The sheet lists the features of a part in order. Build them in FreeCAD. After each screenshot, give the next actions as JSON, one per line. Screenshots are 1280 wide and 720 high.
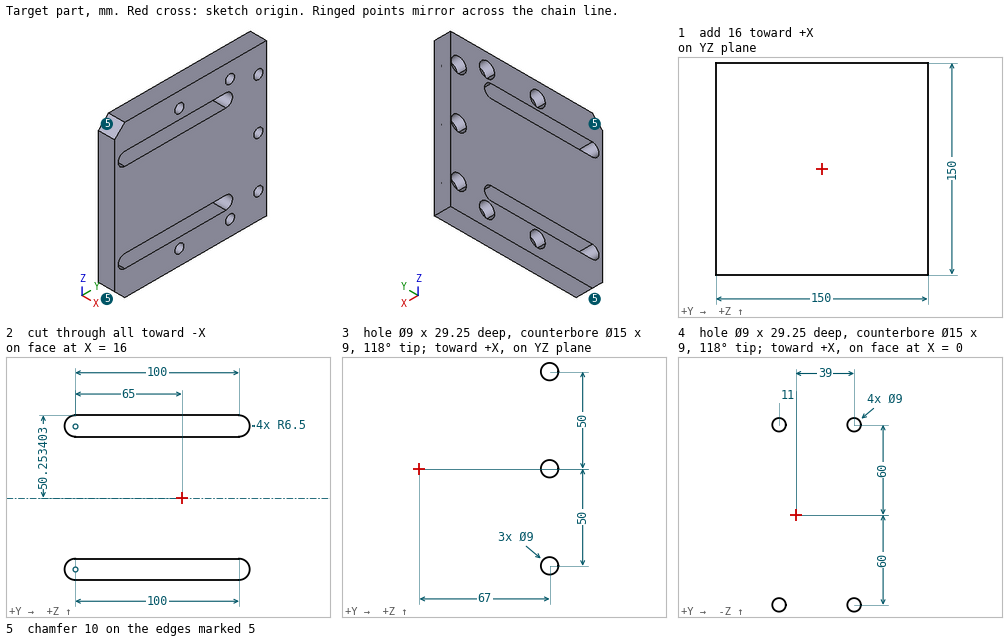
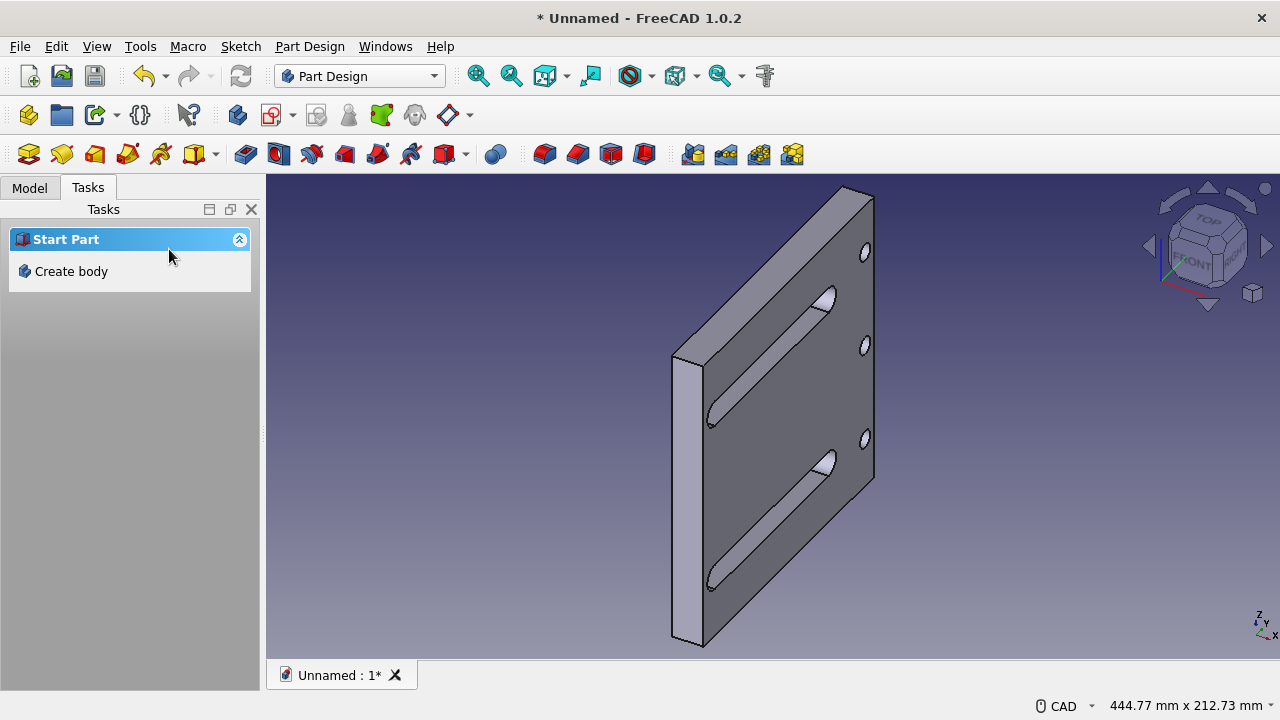
{"action": "key", "text": "6"}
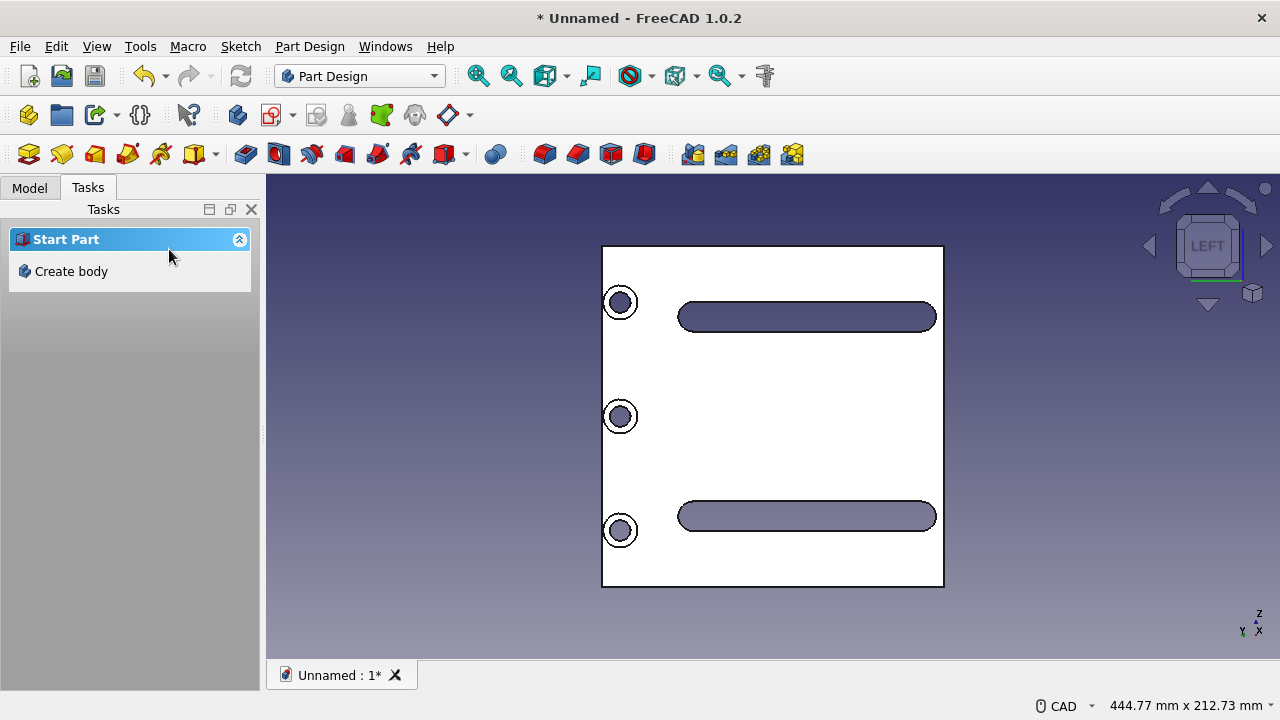
{"action": "left_click", "coordinate": [773, 416]}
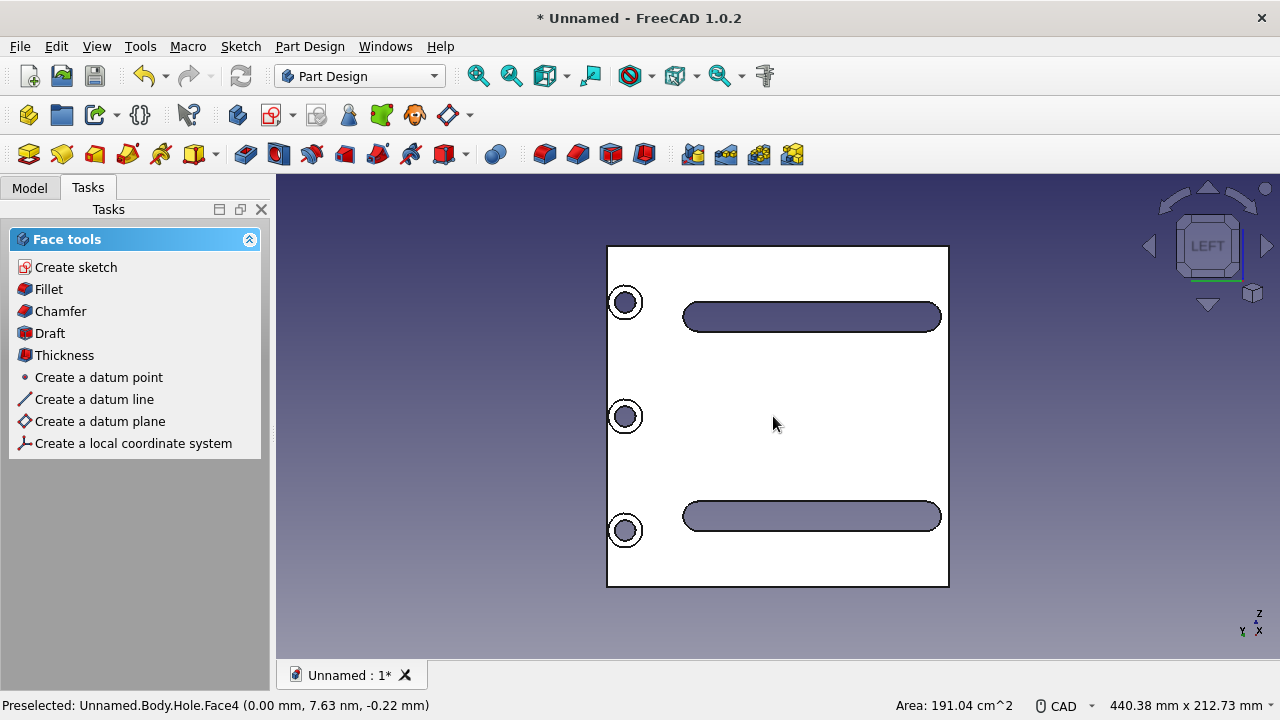
{"action": "left_click", "coordinate": [270, 116]}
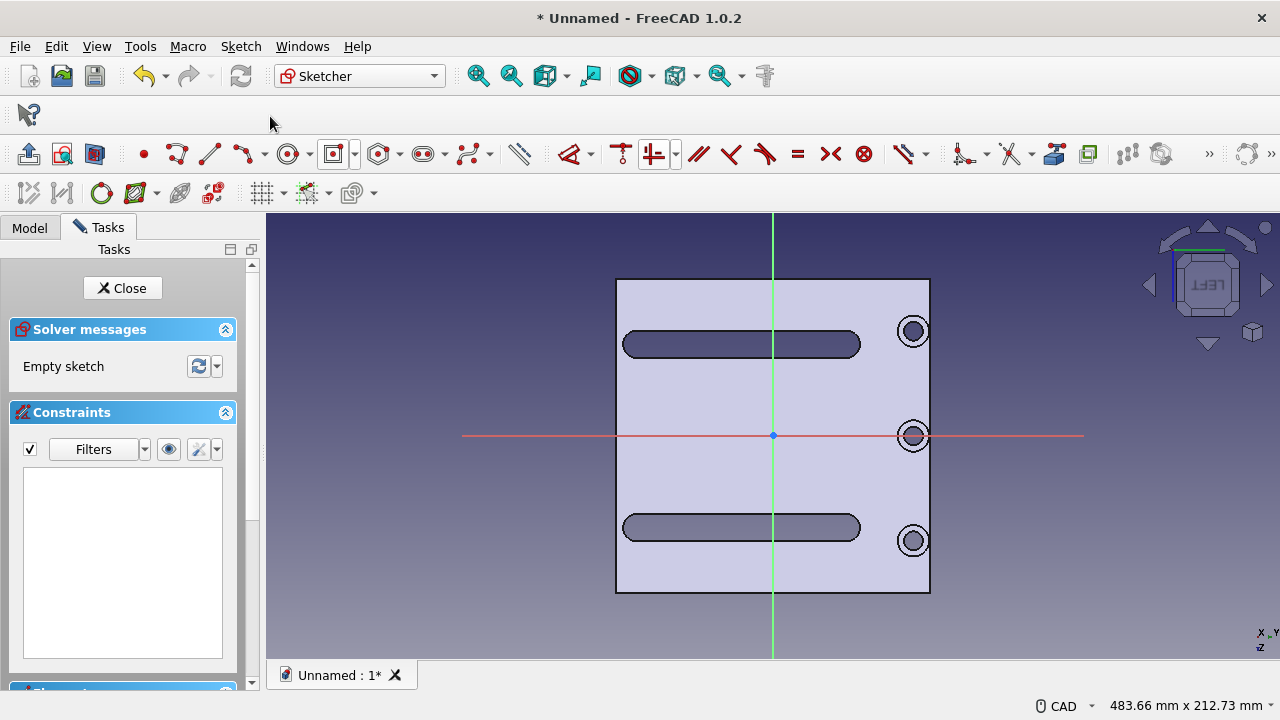
{"action": "key", "text": "g c"}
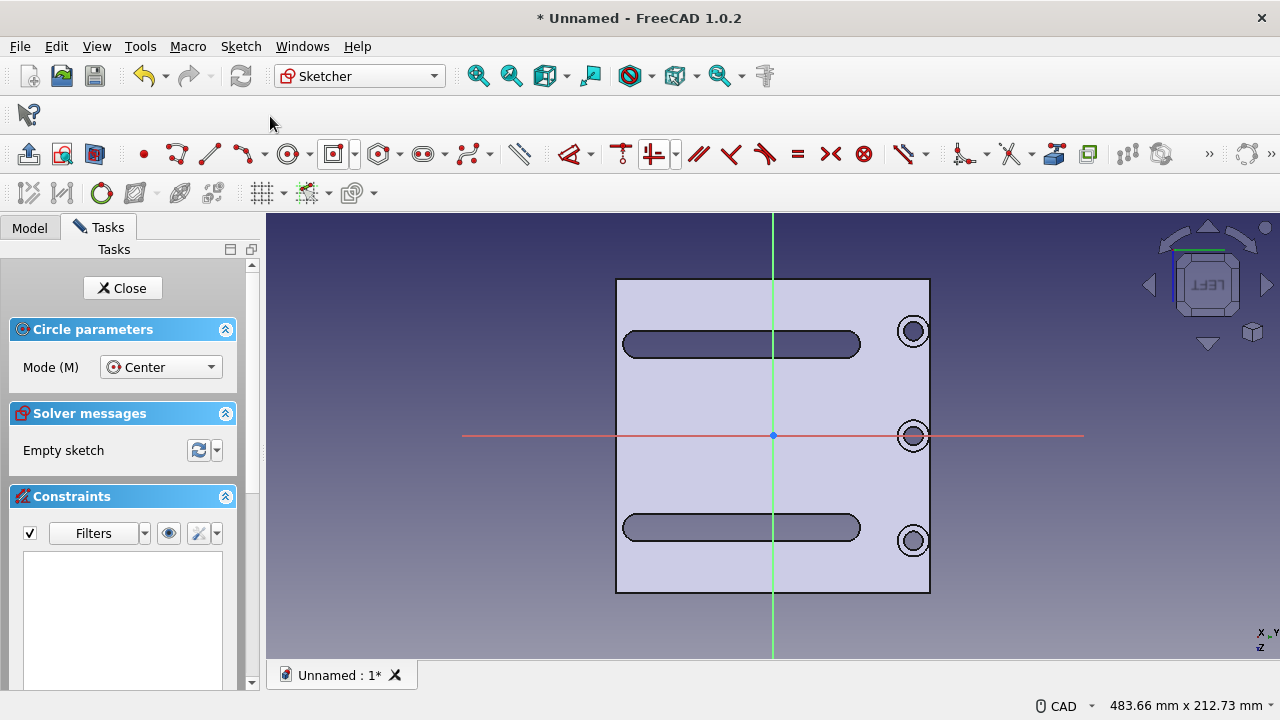
{"action": "scroll", "coordinate": [855, 310], "scroll_direction": "up", "scroll_amount": 5}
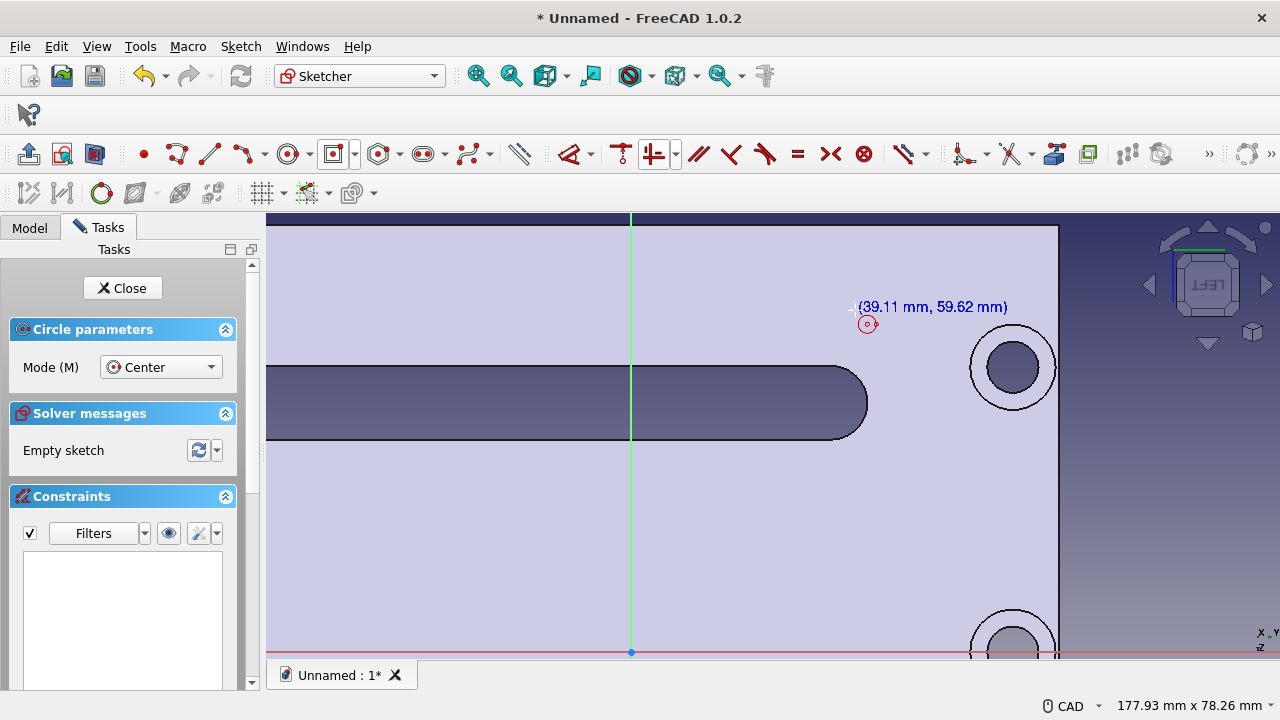
{"action": "left_click", "coordinate": [853, 310]}
{"action": "mouse_move", "coordinate": [871, 292]}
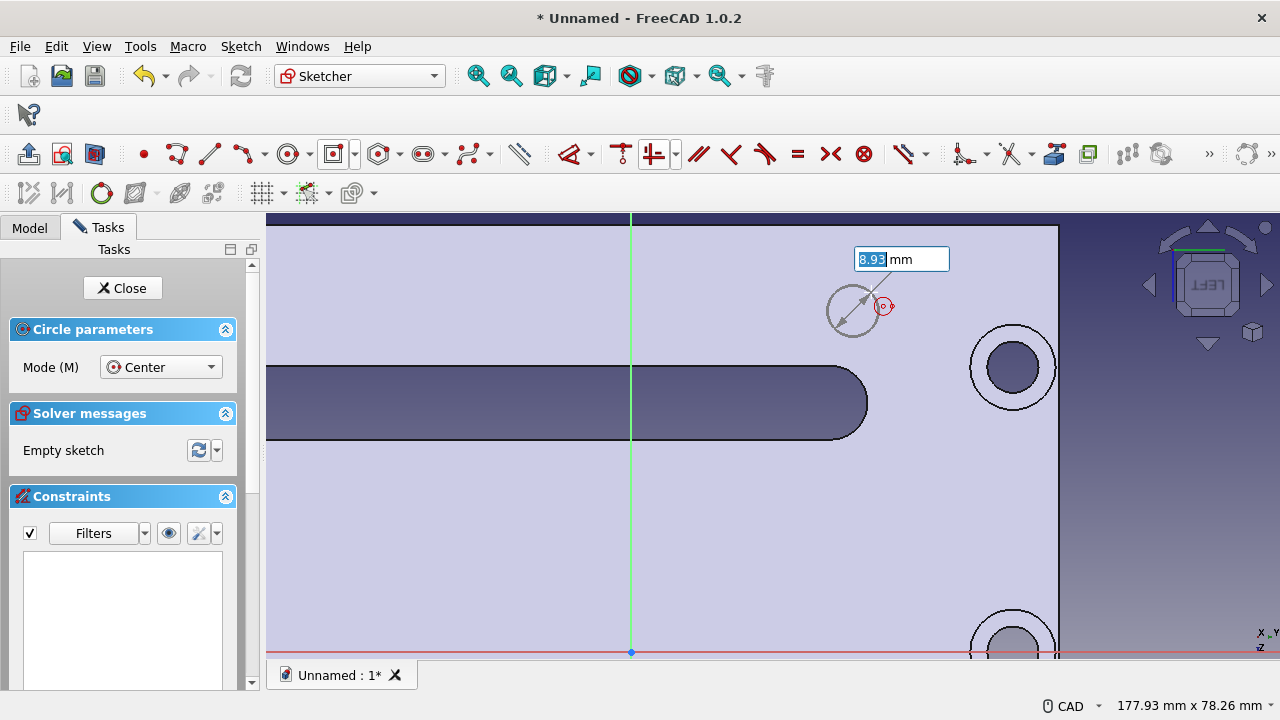
{"action": "type", "text": "9"}
{"action": "key", "text": "Return"}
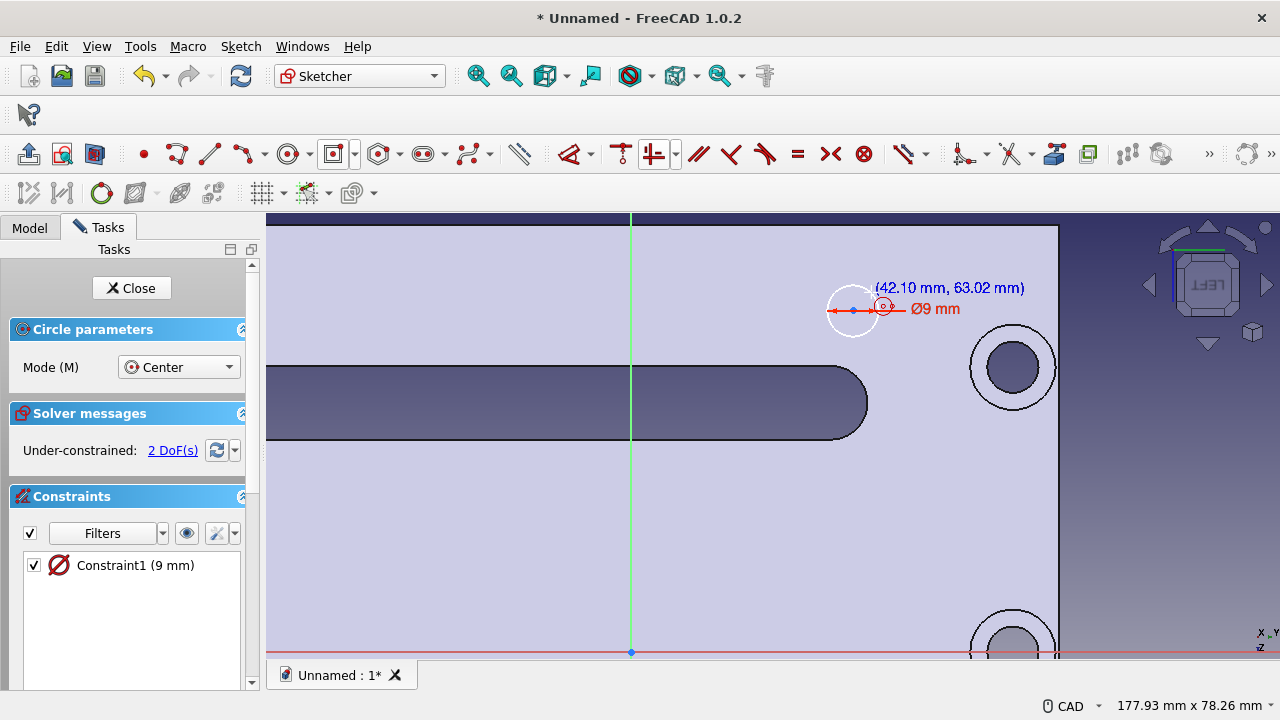
{"action": "left_click", "coordinate": [568, 310]}
{"action": "mouse_move", "coordinate": [587, 292]}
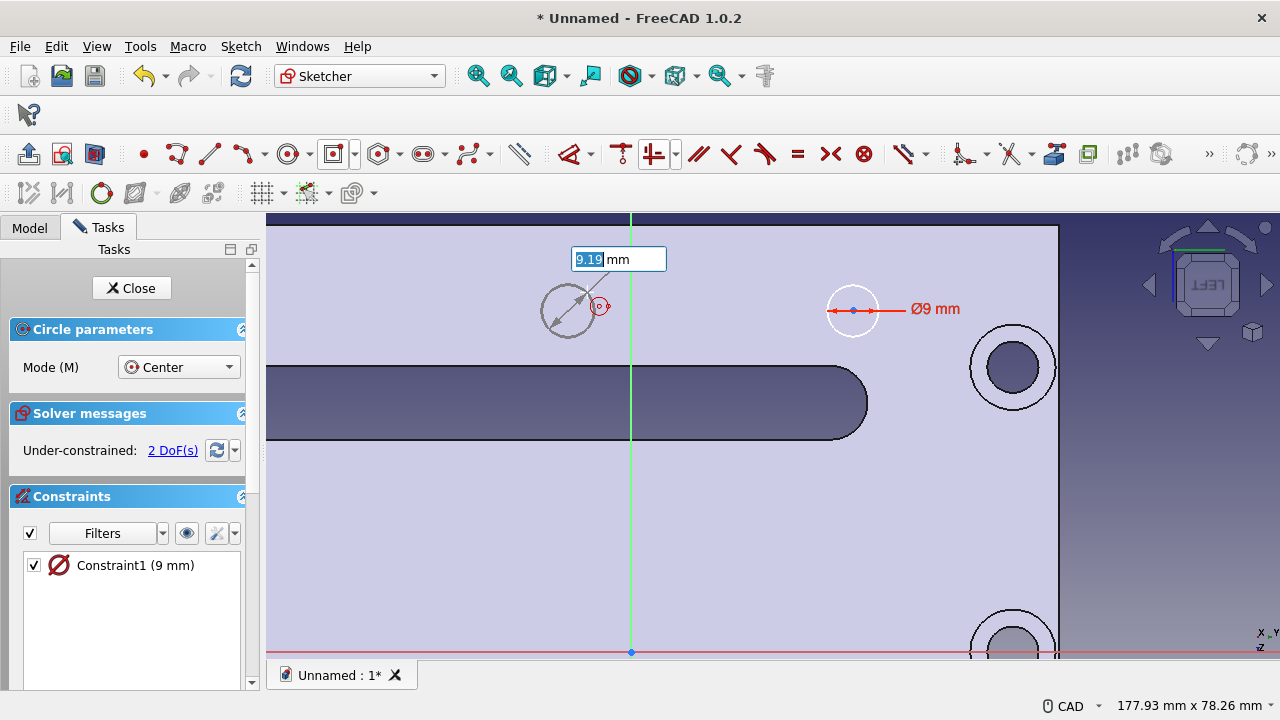
{"action": "type", "text": "9"}
{"action": "key", "text": "Return"}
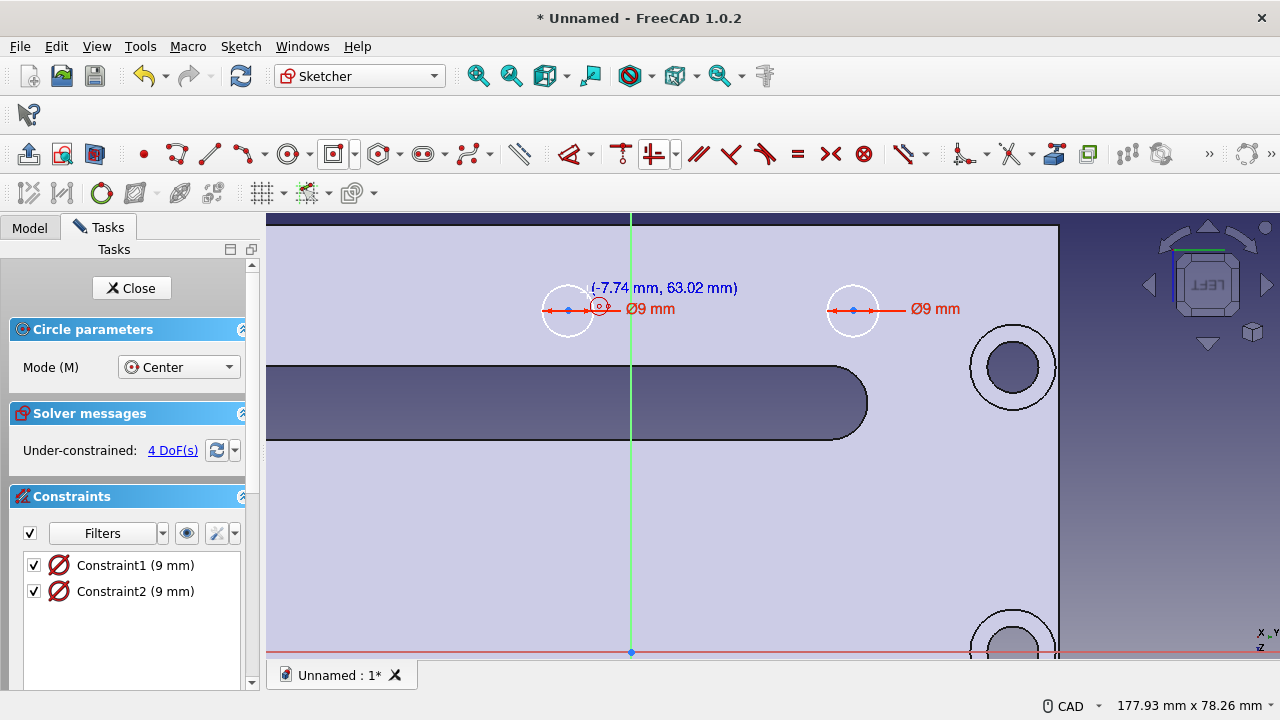
{"action": "scroll", "coordinate": [701, 310], "scroll_direction": "down", "scroll_amount": 5}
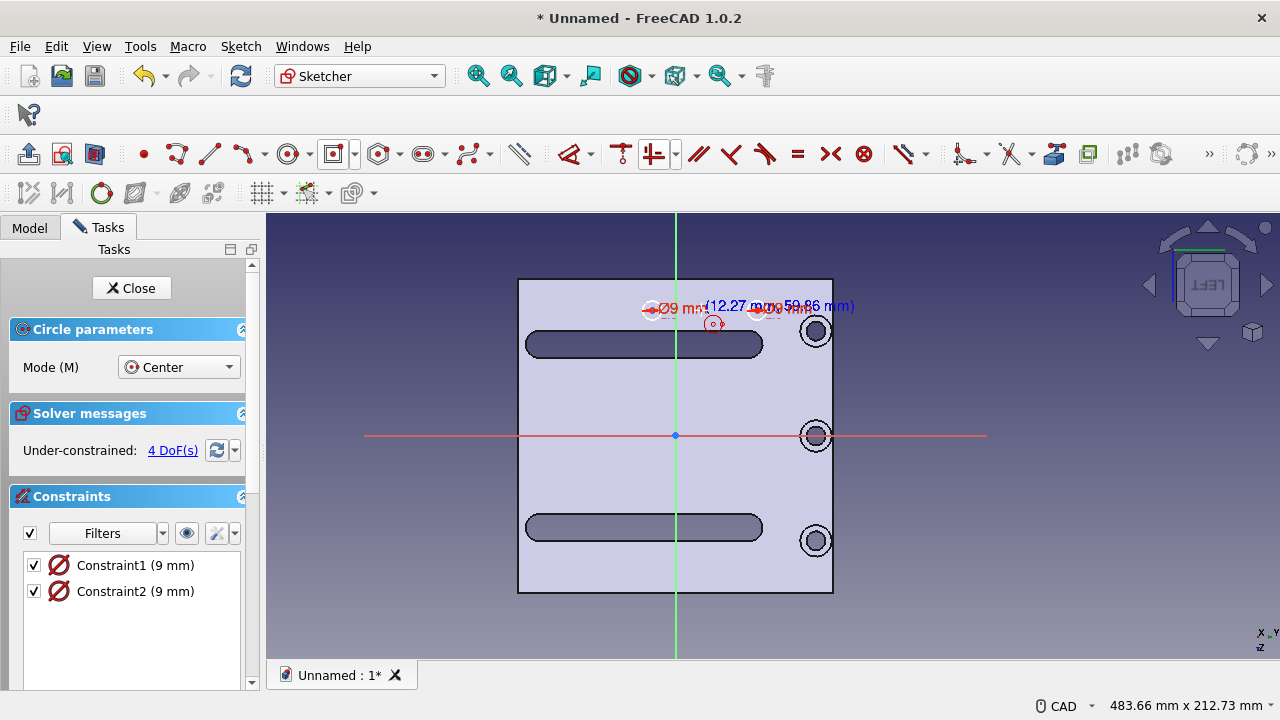
{"action": "scroll", "coordinate": [757, 562], "scroll_direction": "up", "scroll_amount": 5}